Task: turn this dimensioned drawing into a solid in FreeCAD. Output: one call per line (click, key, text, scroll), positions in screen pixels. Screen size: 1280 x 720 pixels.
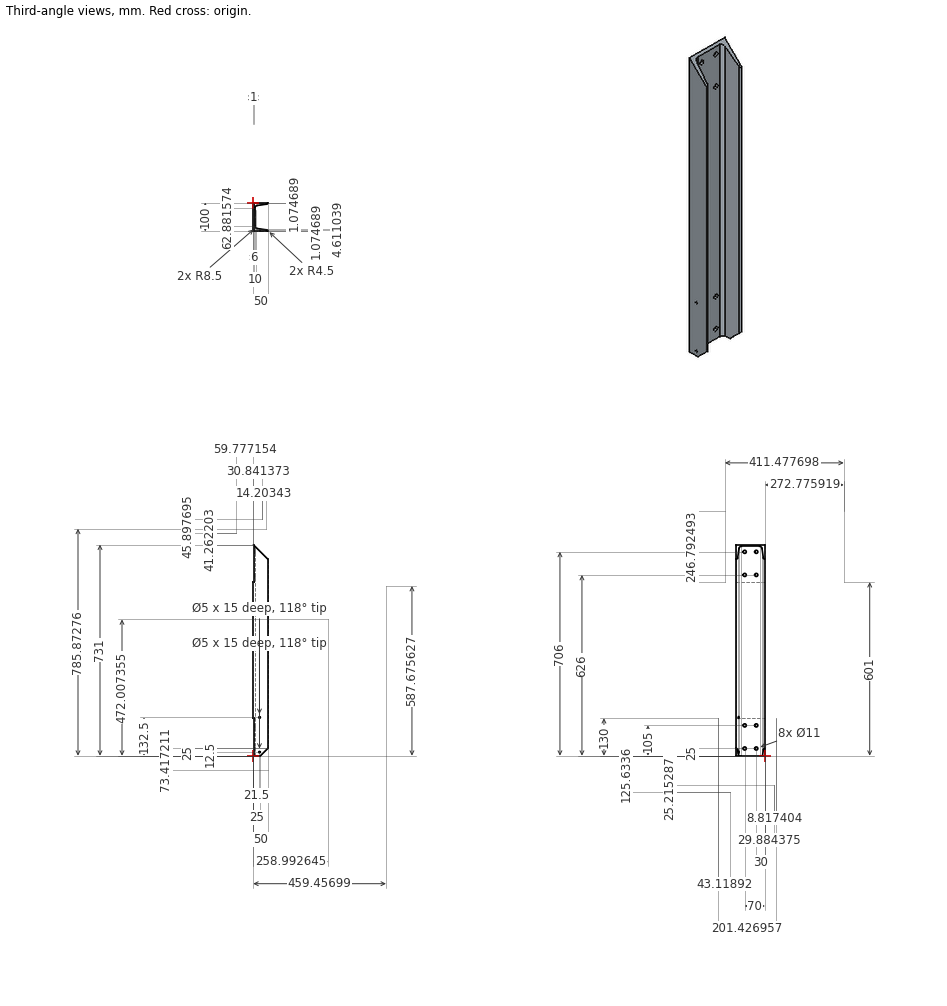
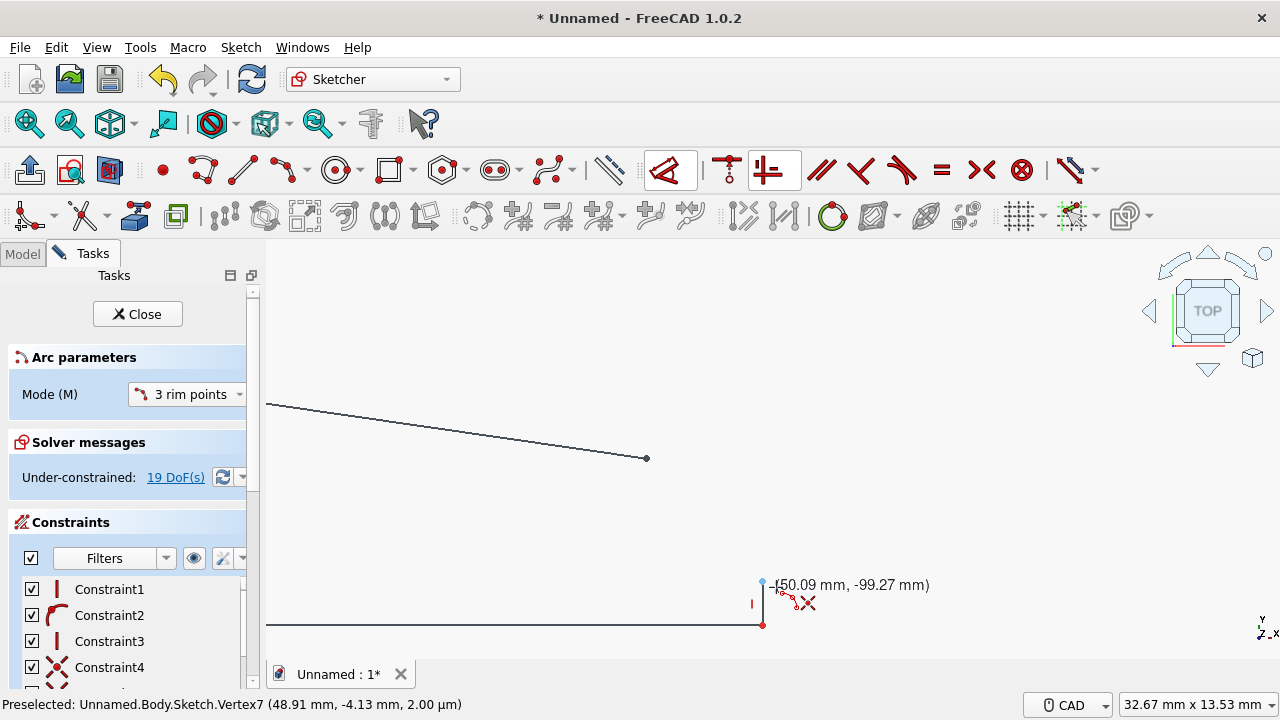
click(763, 581)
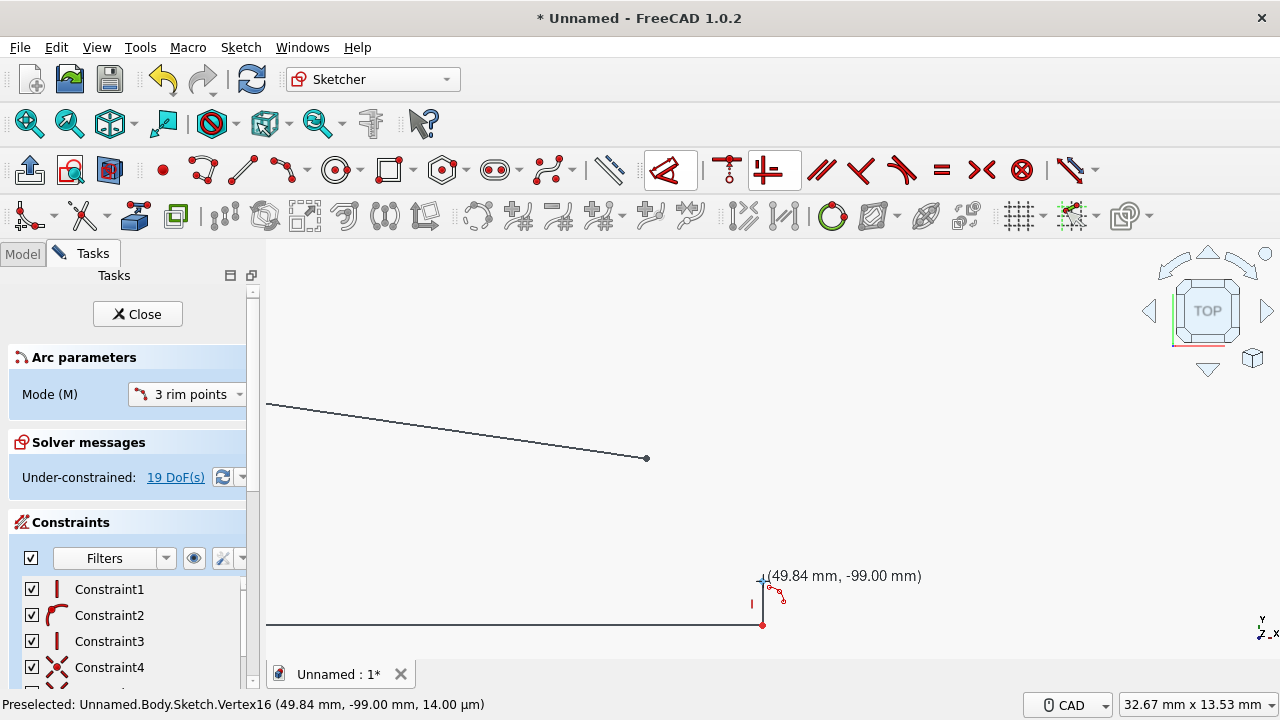
scroll(776, 588, down, 12)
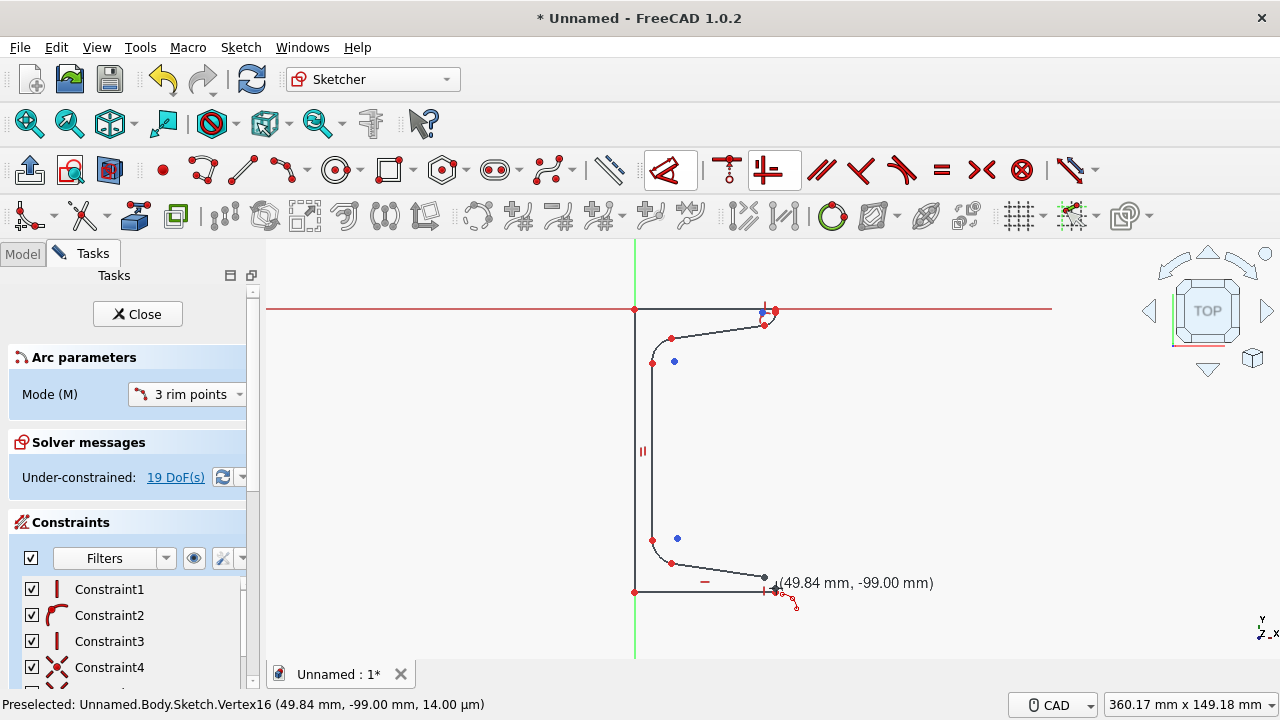
click(765, 577)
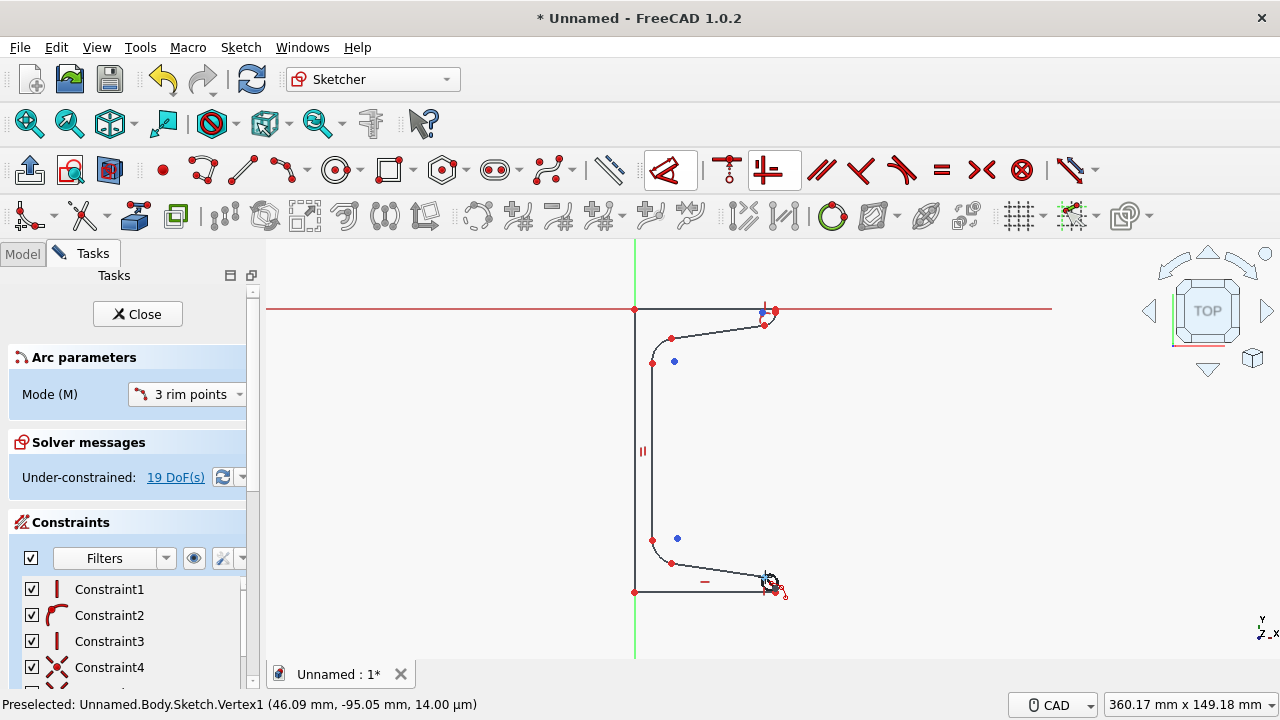
scroll(773, 580, up, 9)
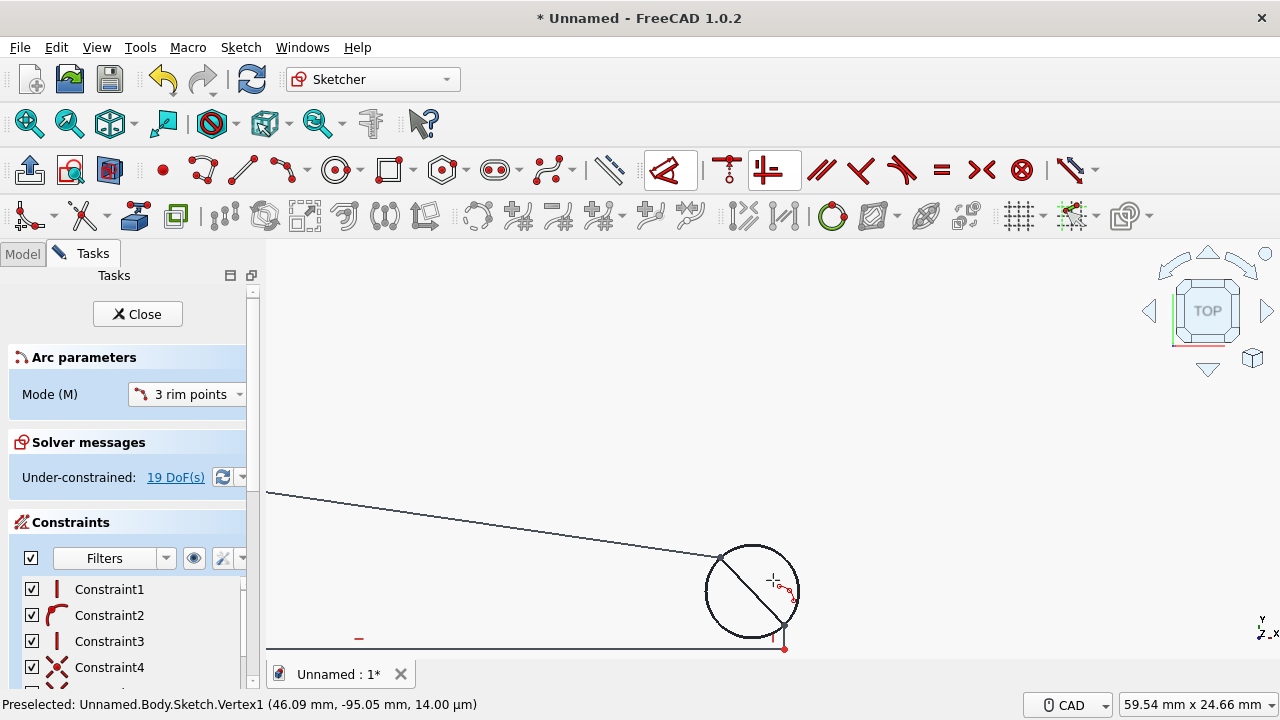
click(768, 574)
key(Escape)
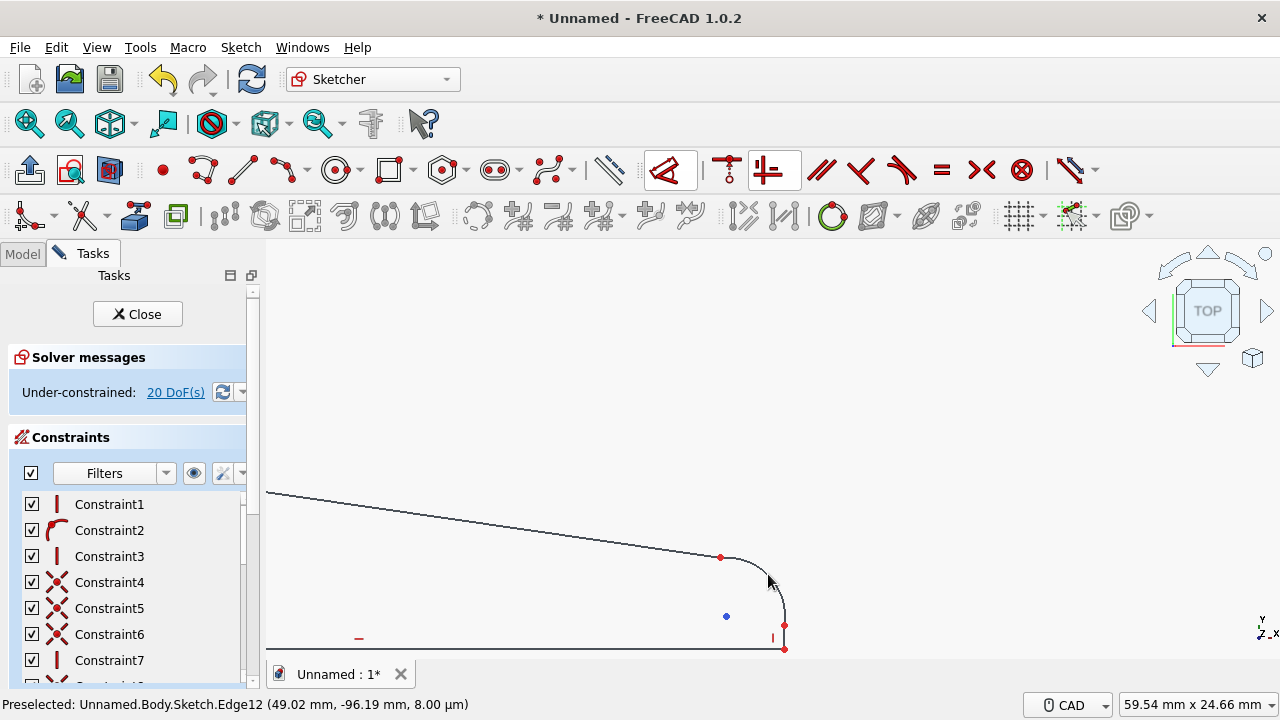
scroll(772, 579, down, 9)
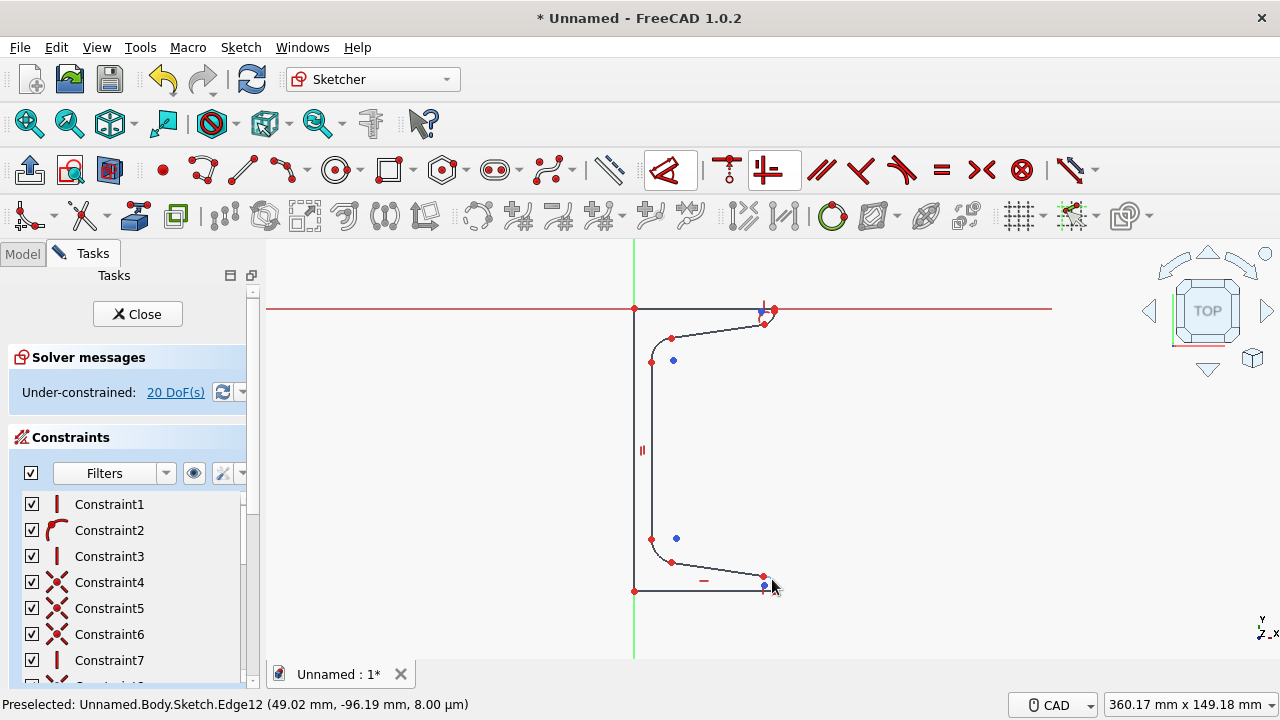
click(736, 572)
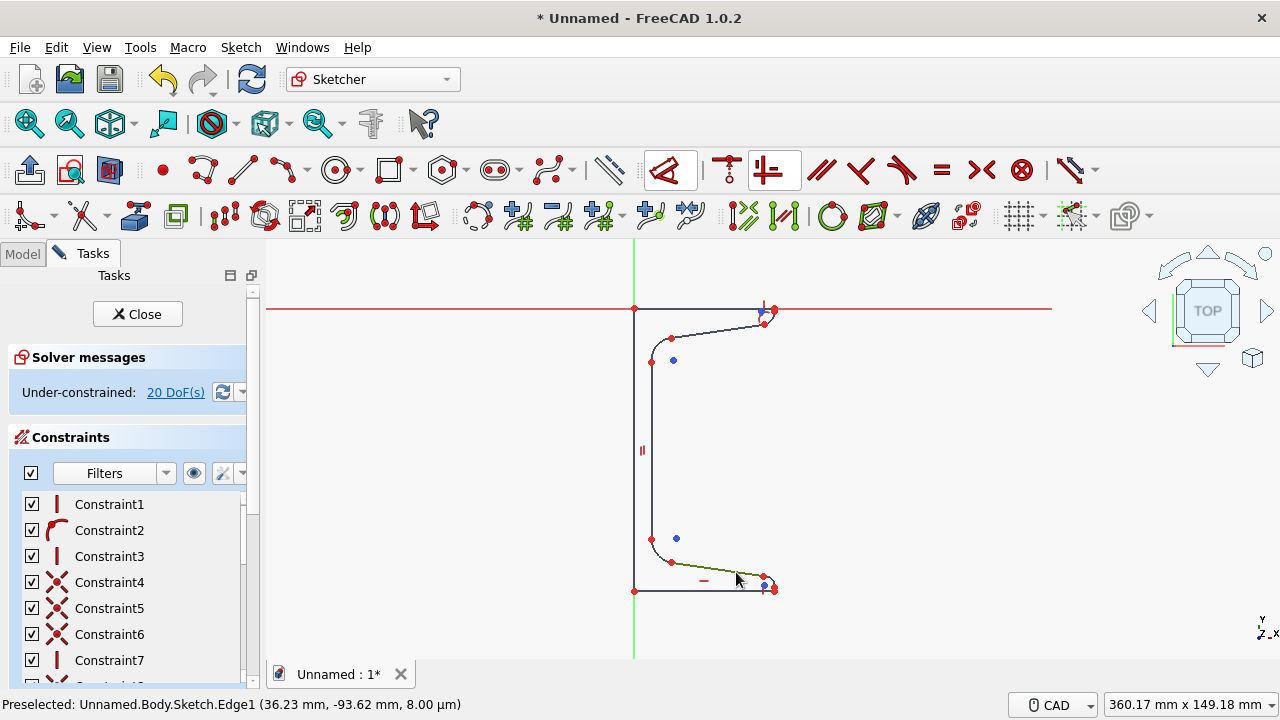
scroll(654, 549, up, 2)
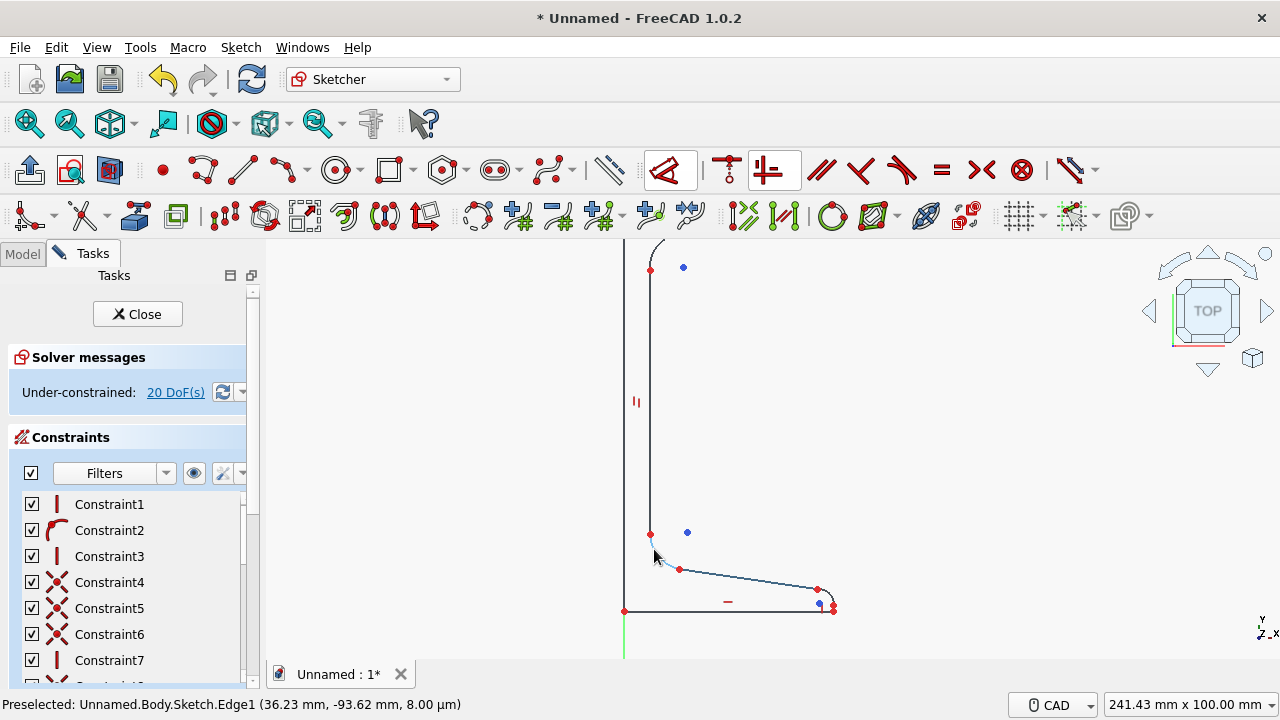
click(654, 549)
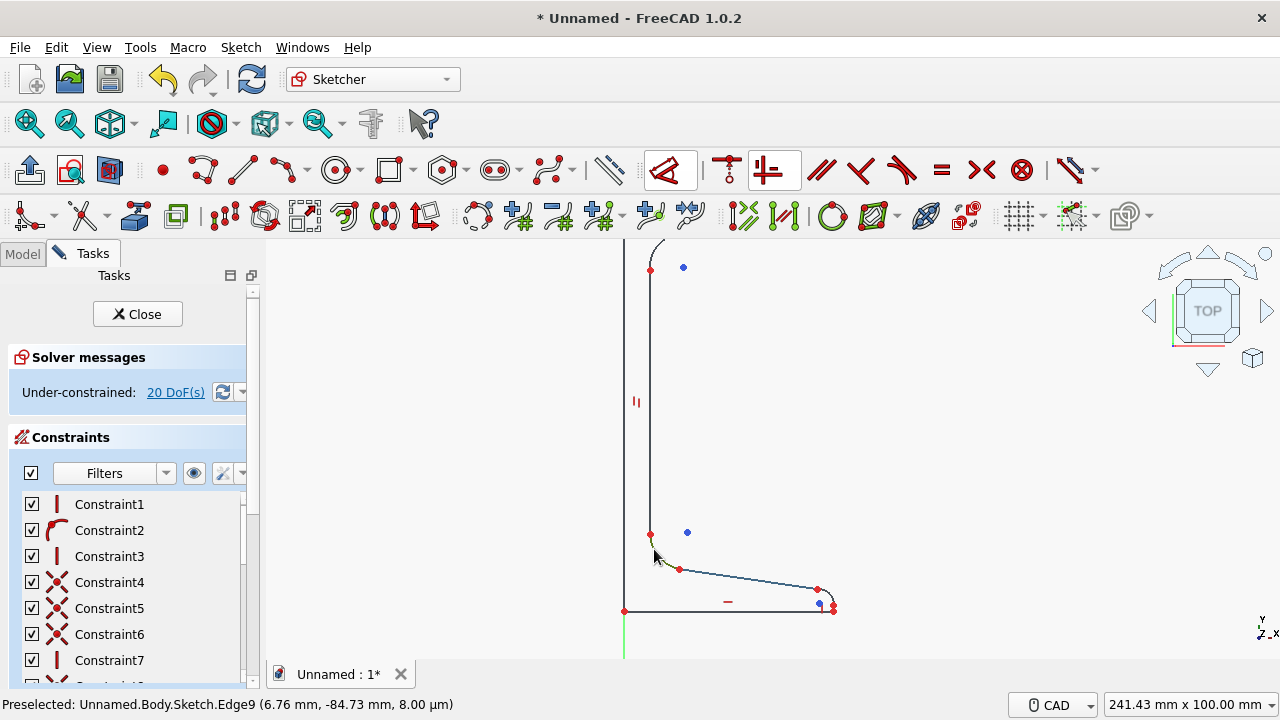
click(902, 170)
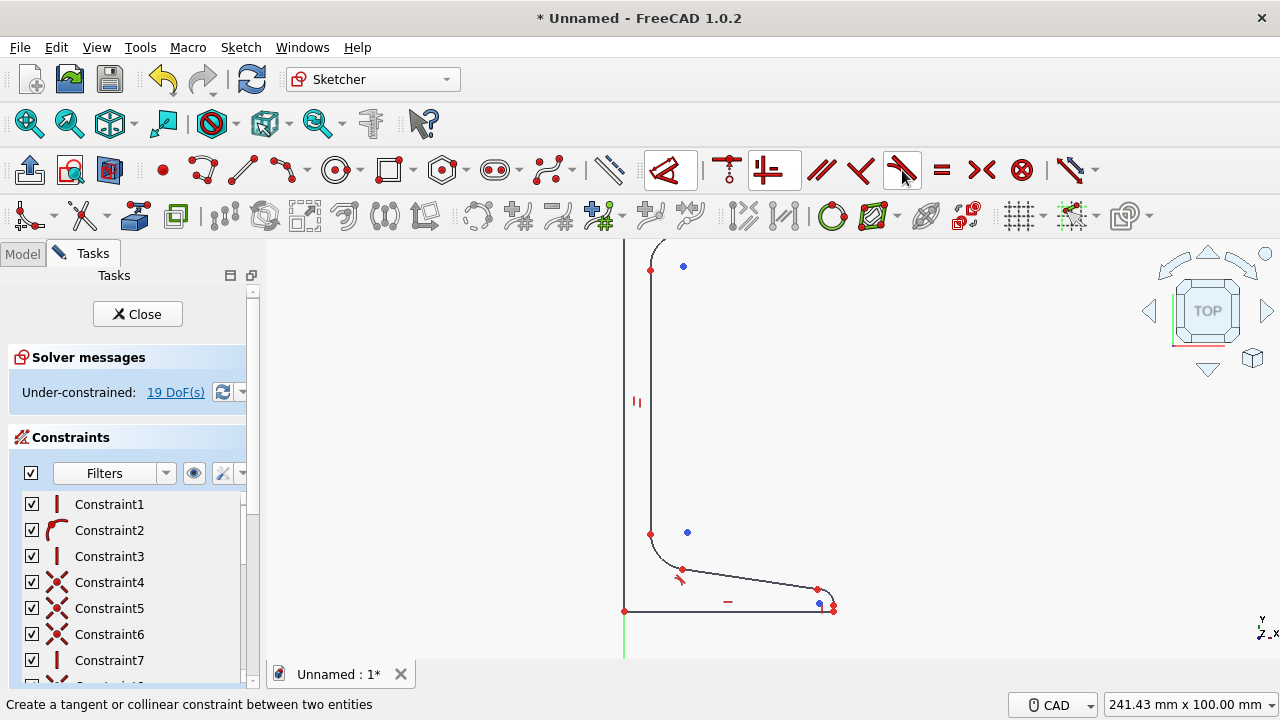
click(777, 583)